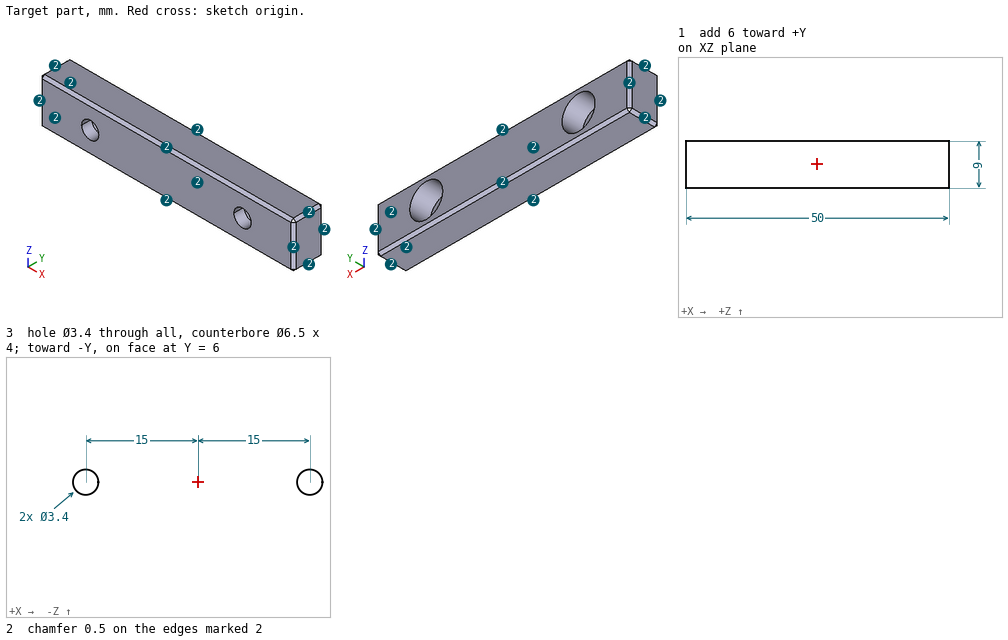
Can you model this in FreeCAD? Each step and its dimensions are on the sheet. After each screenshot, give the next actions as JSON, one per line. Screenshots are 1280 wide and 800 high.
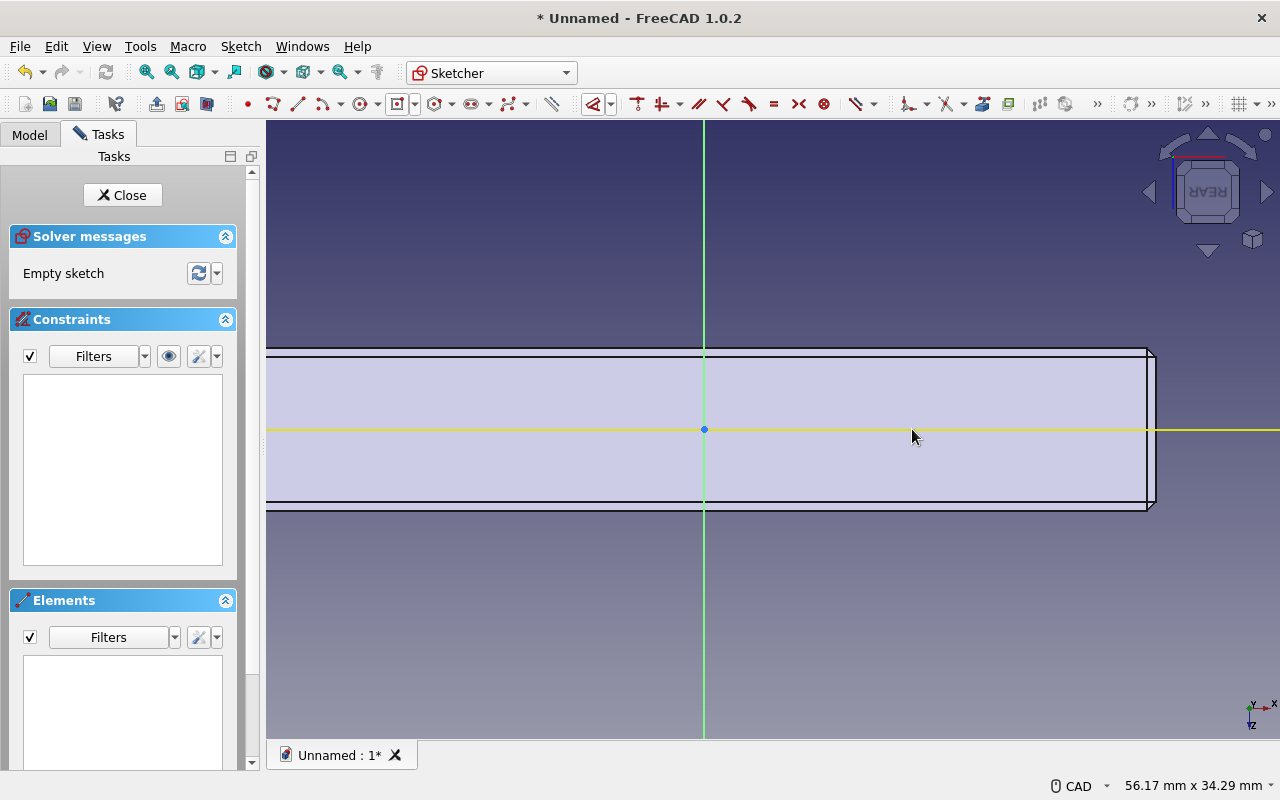
{"action": "left_click", "coordinate": [360, 104]}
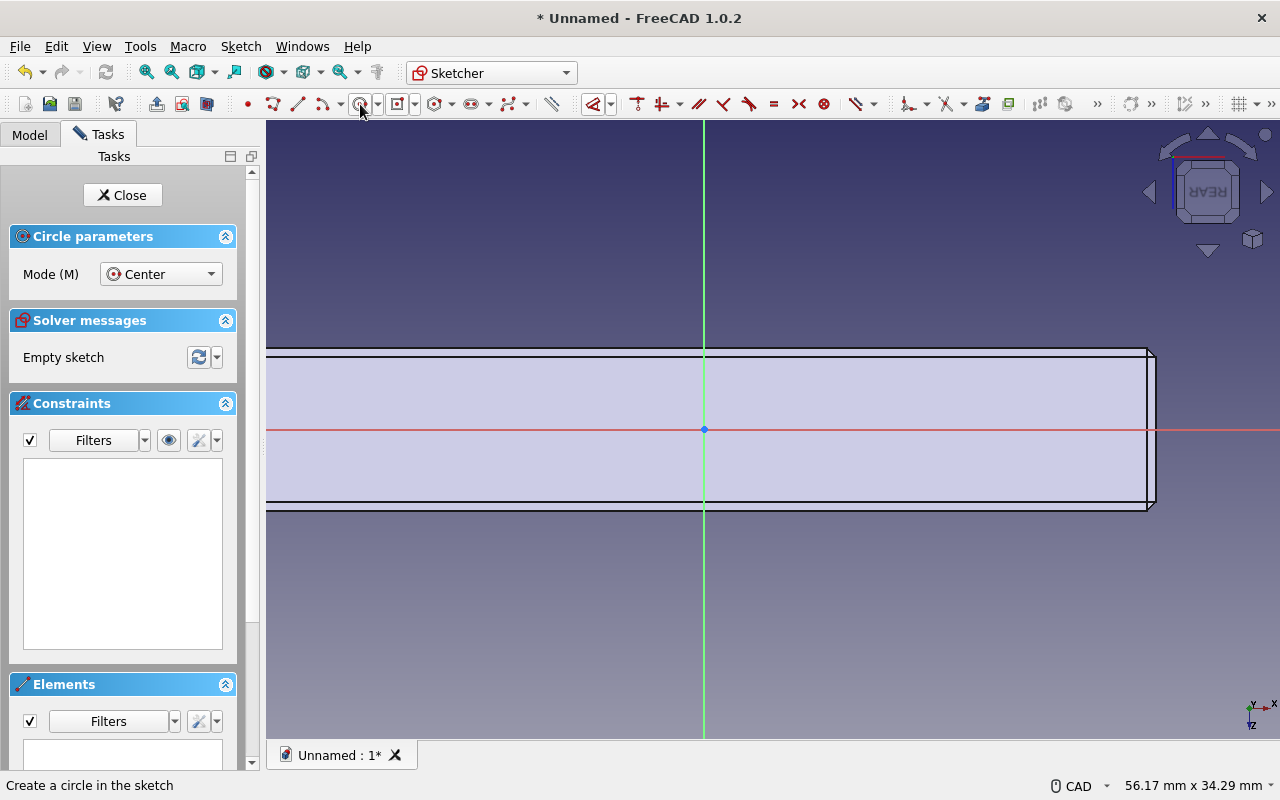
{"action": "left_click", "coordinate": [434, 429]}
{"action": "left_click", "coordinate": [455, 408]}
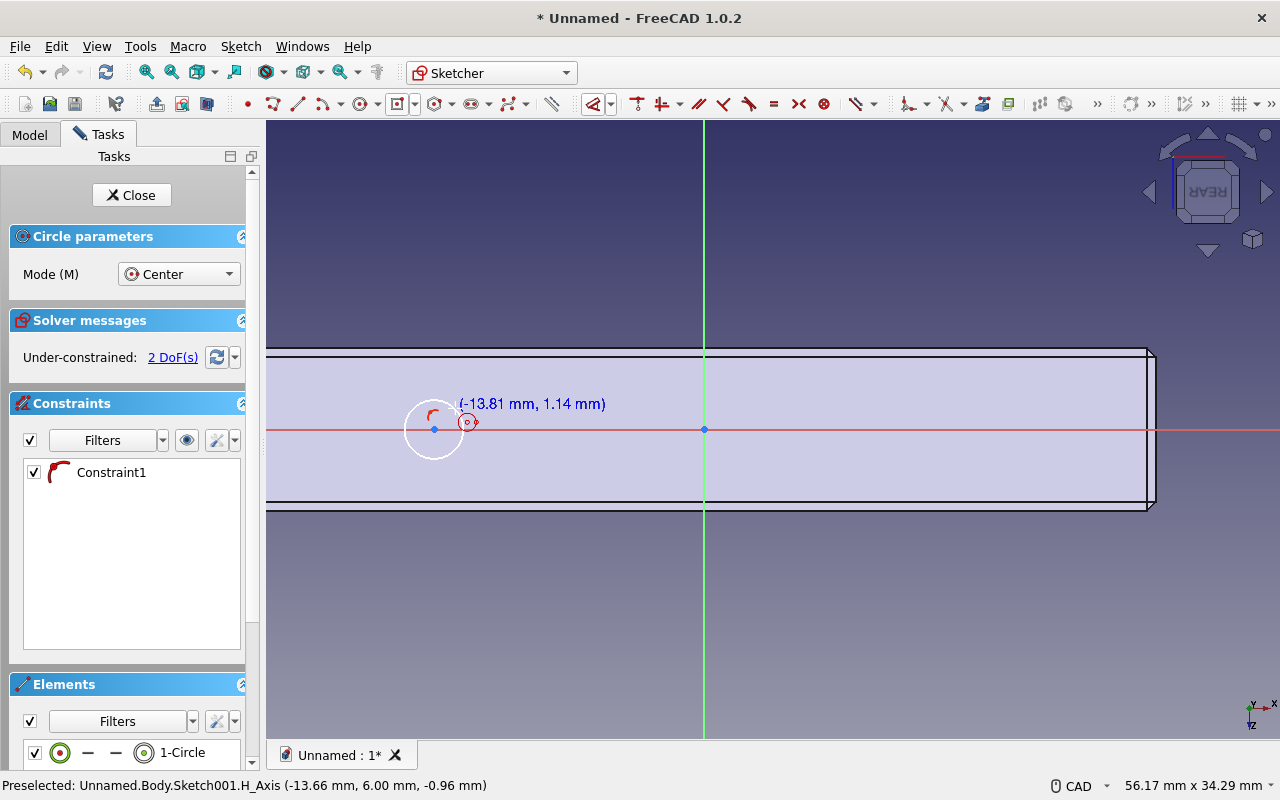
{"action": "left_click", "coordinate": [975, 429]}
{"action": "left_click", "coordinate": [997, 408]}
{"action": "key", "text": "Escape"}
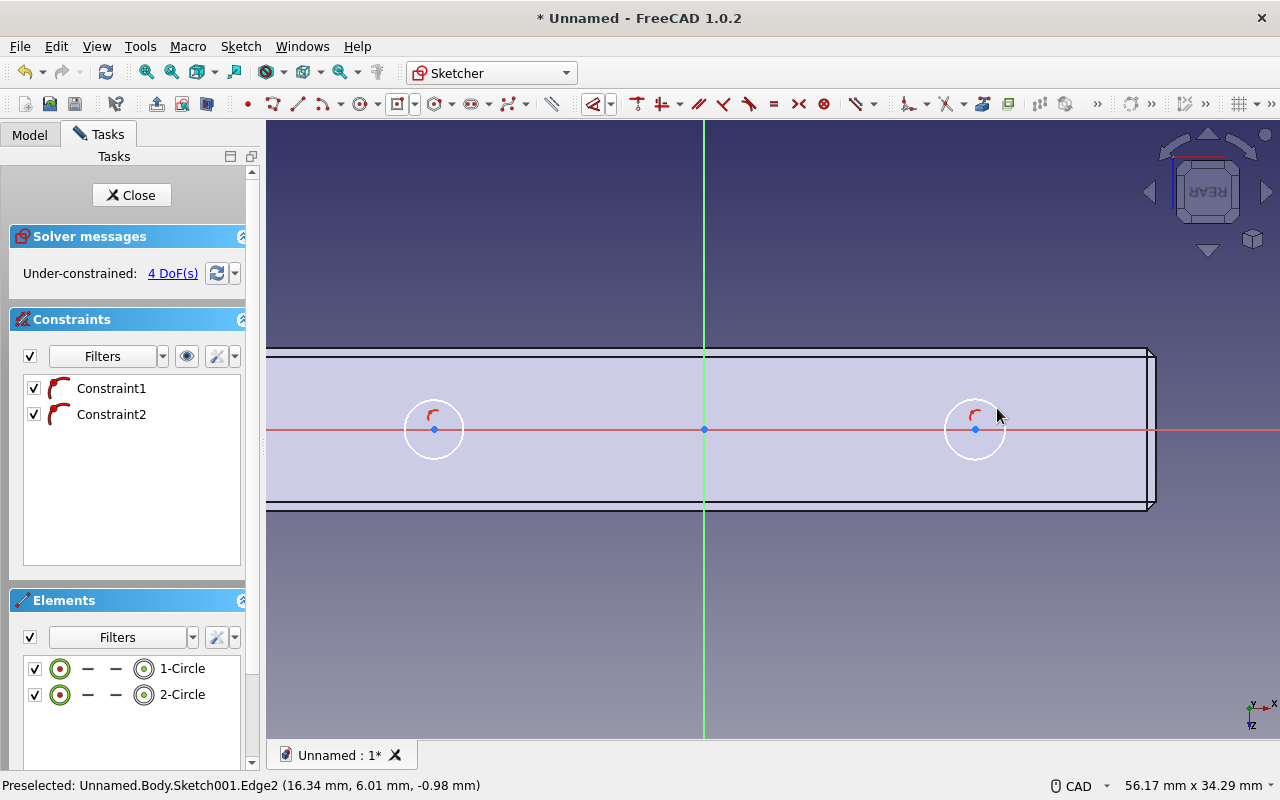
{"action": "left_click", "coordinate": [455, 409]}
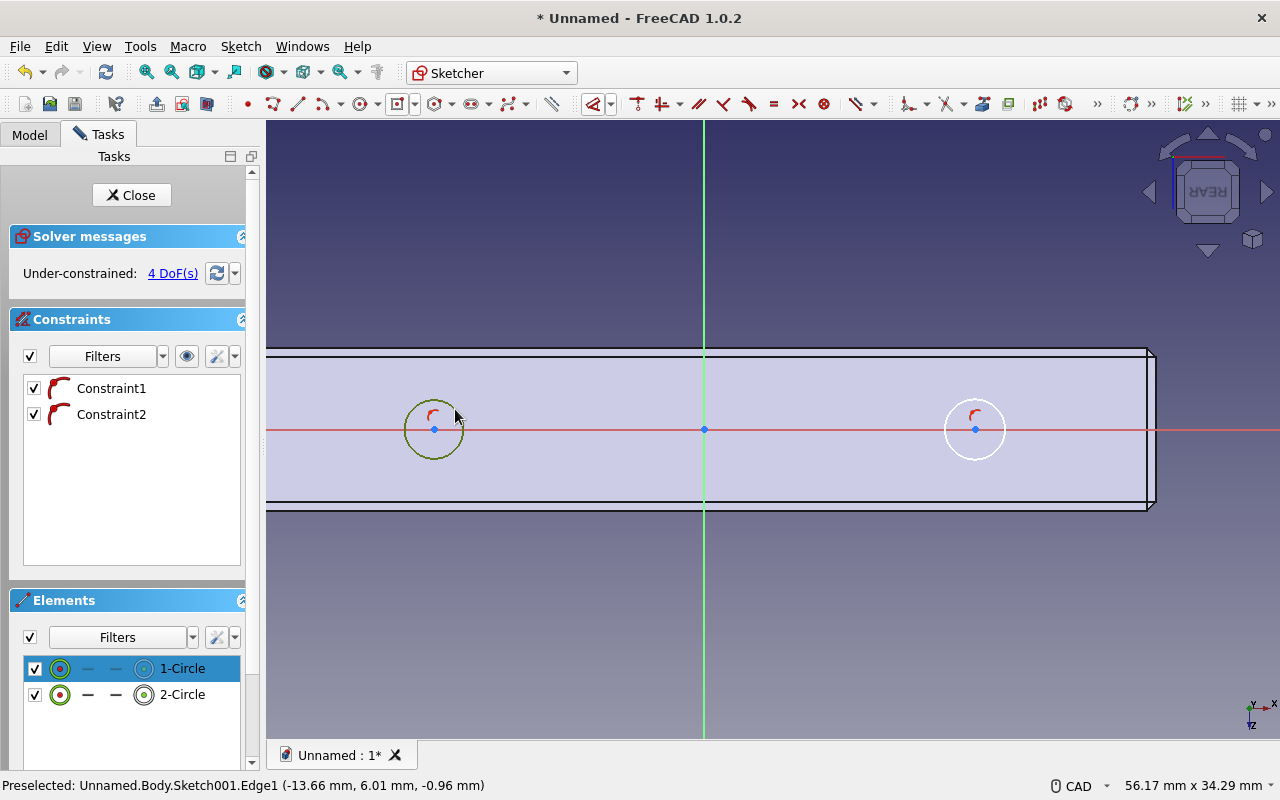
{"action": "left_click", "coordinate": [996, 408]}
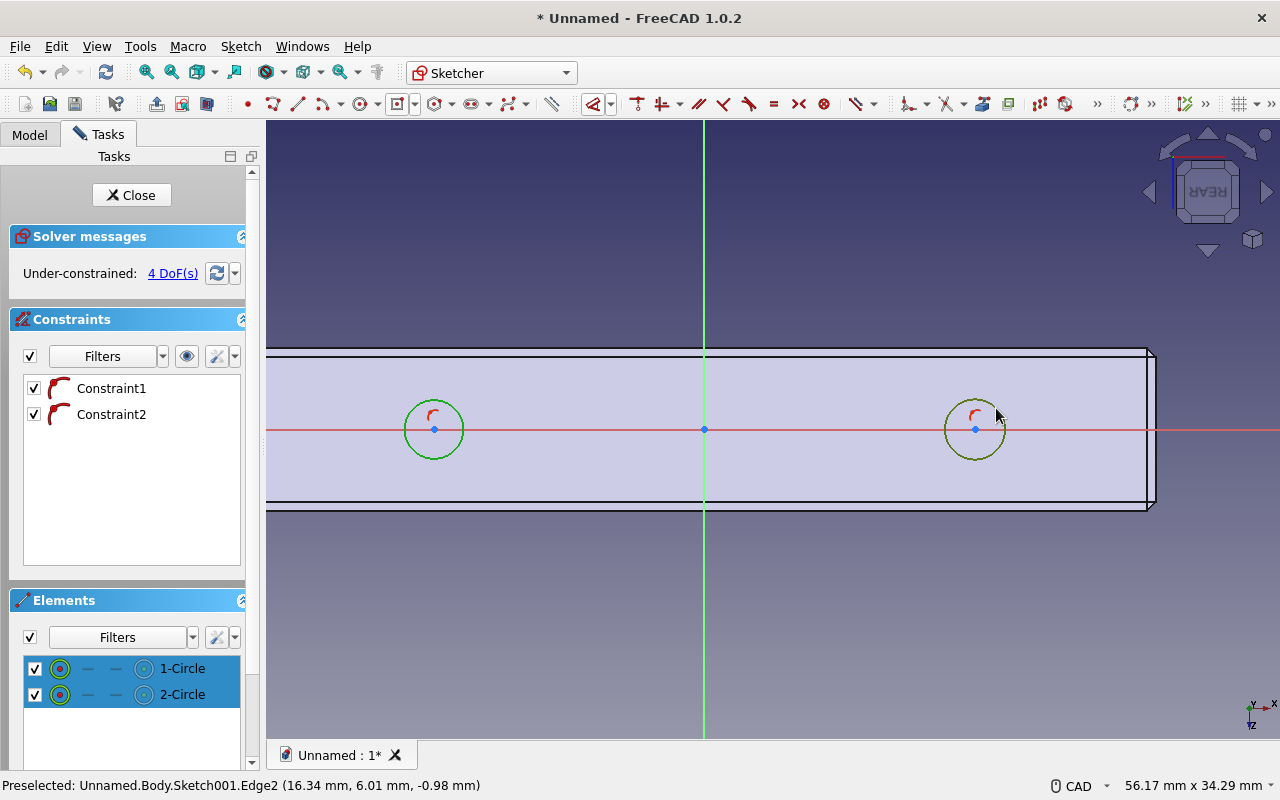
{"action": "left_click", "coordinate": [774, 104]}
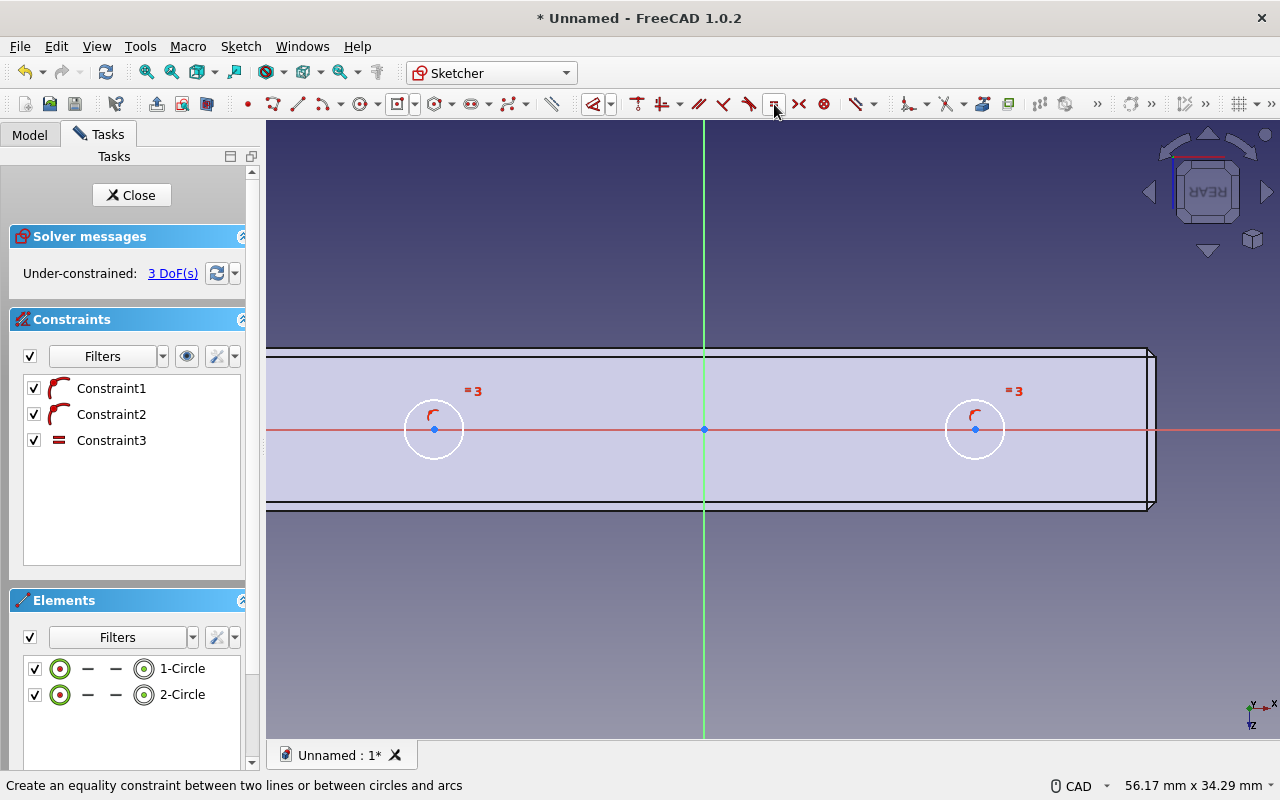
{"action": "left_click", "coordinate": [455, 409]}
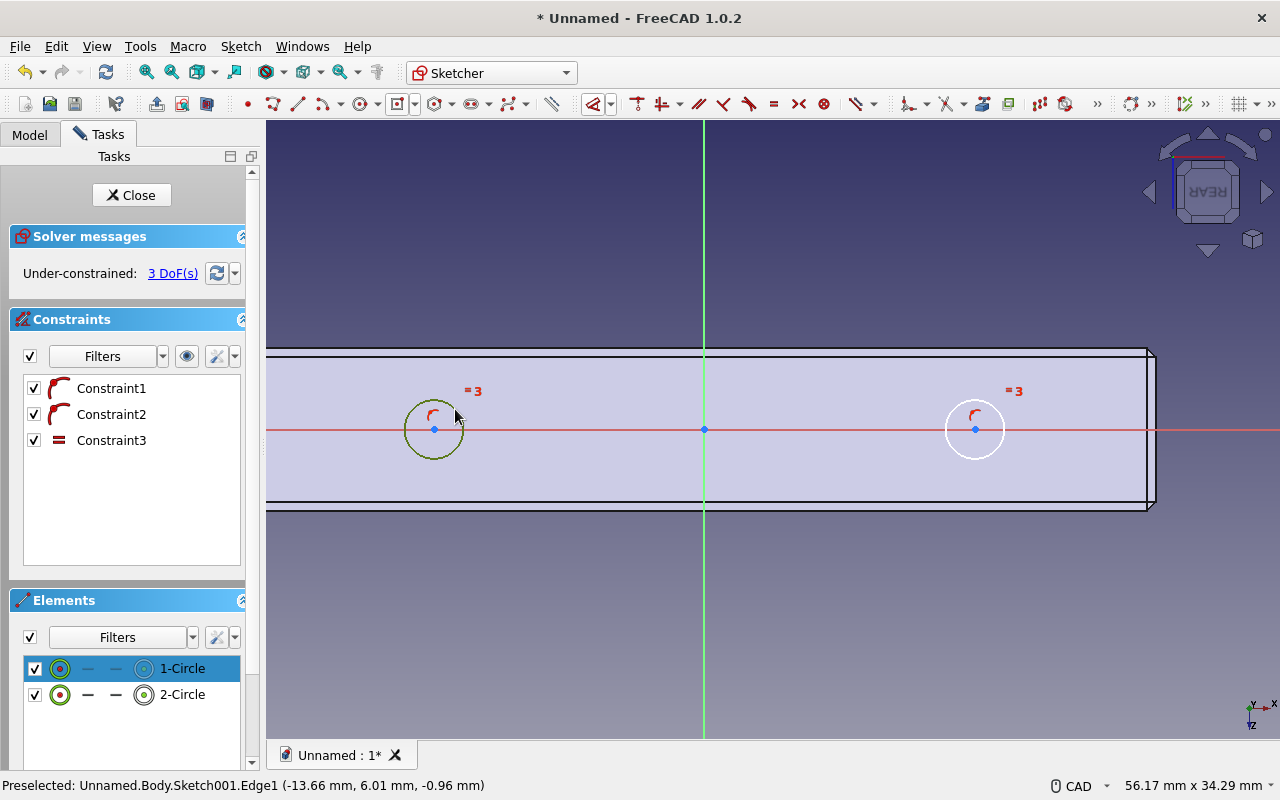
{"action": "key", "text": "k o"}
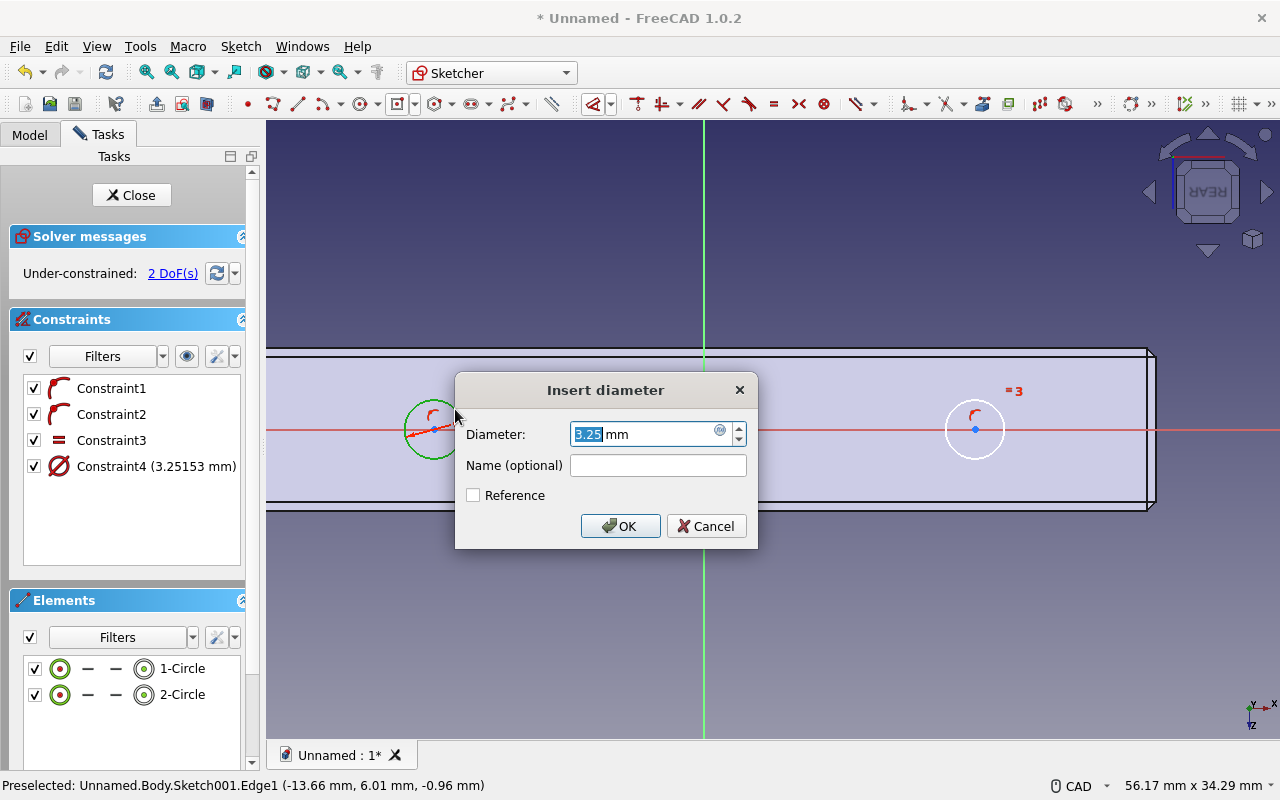
{"action": "type", "text": "3.4"}
{"action": "key", "text": "Return"}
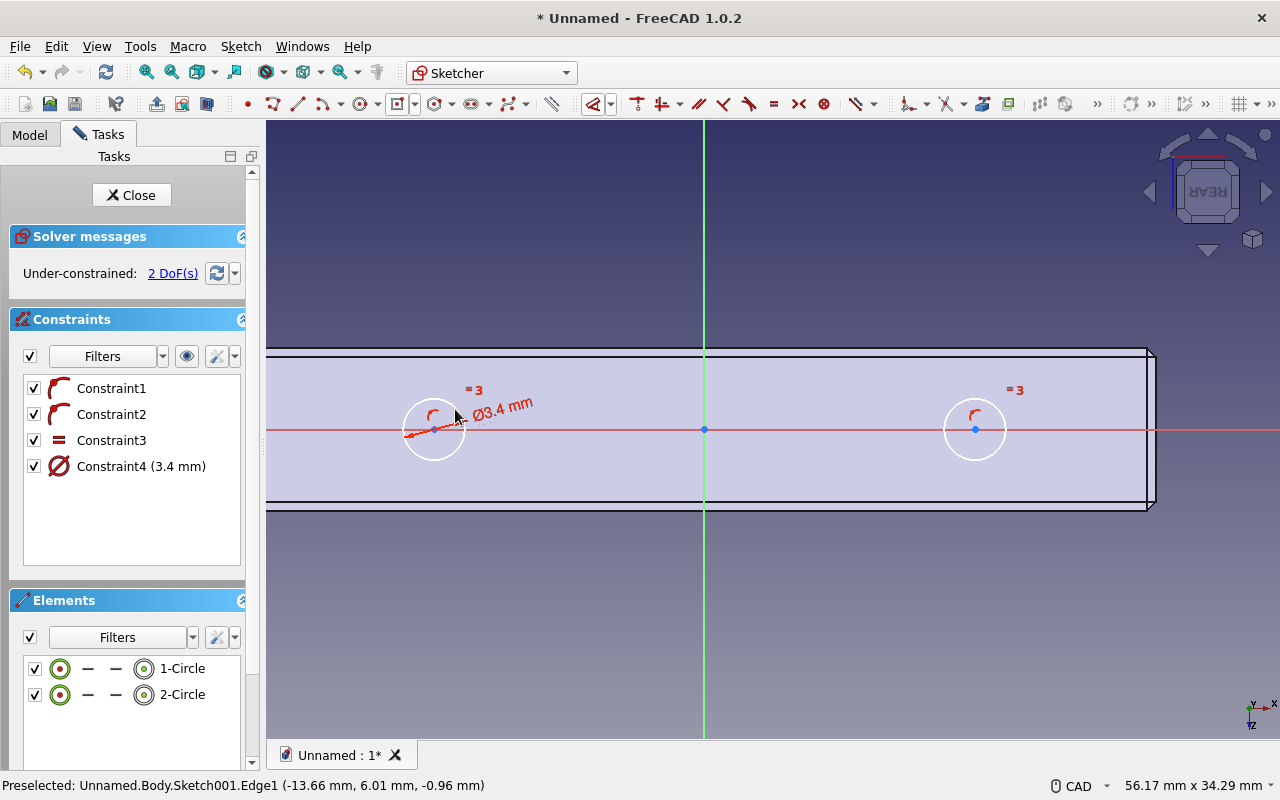
{"action": "left_click", "coordinate": [434, 429]}